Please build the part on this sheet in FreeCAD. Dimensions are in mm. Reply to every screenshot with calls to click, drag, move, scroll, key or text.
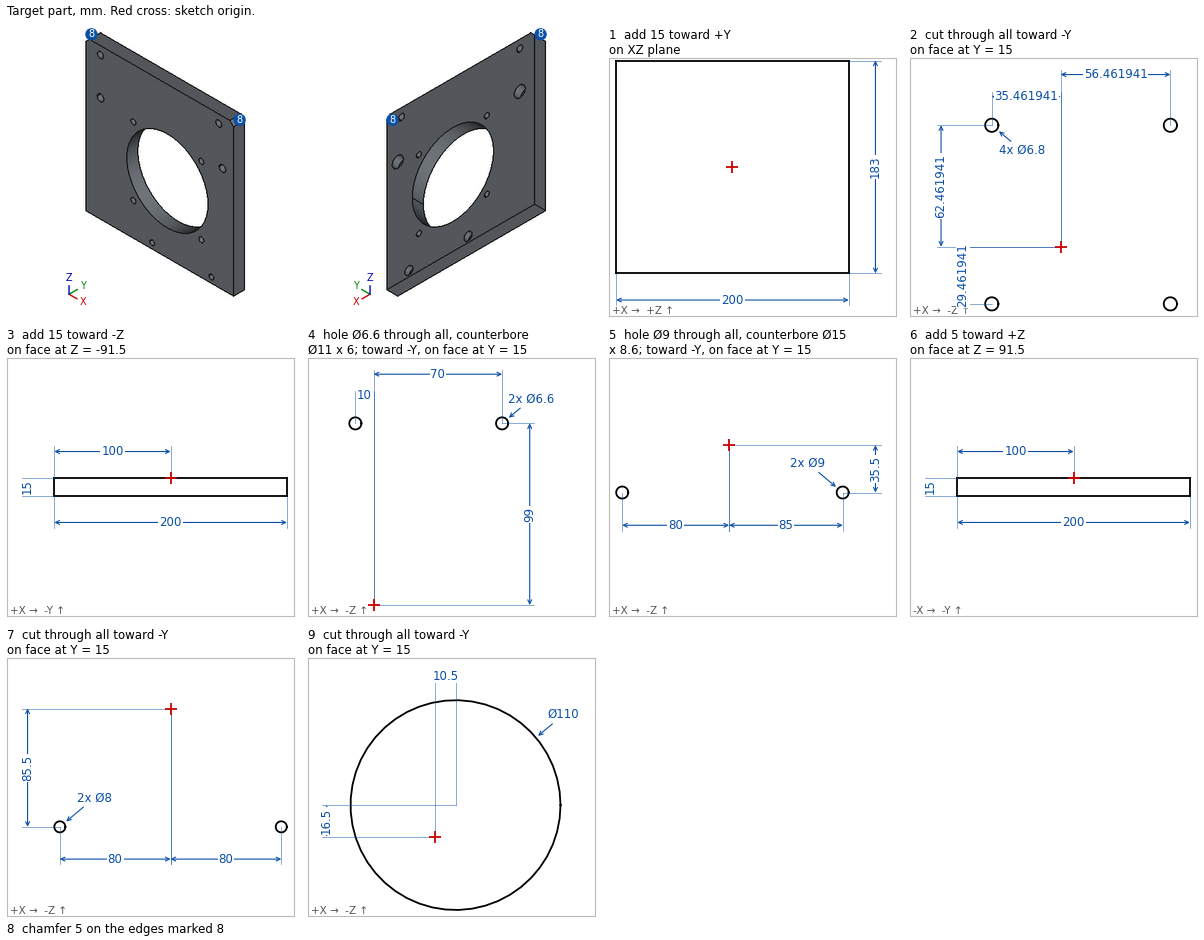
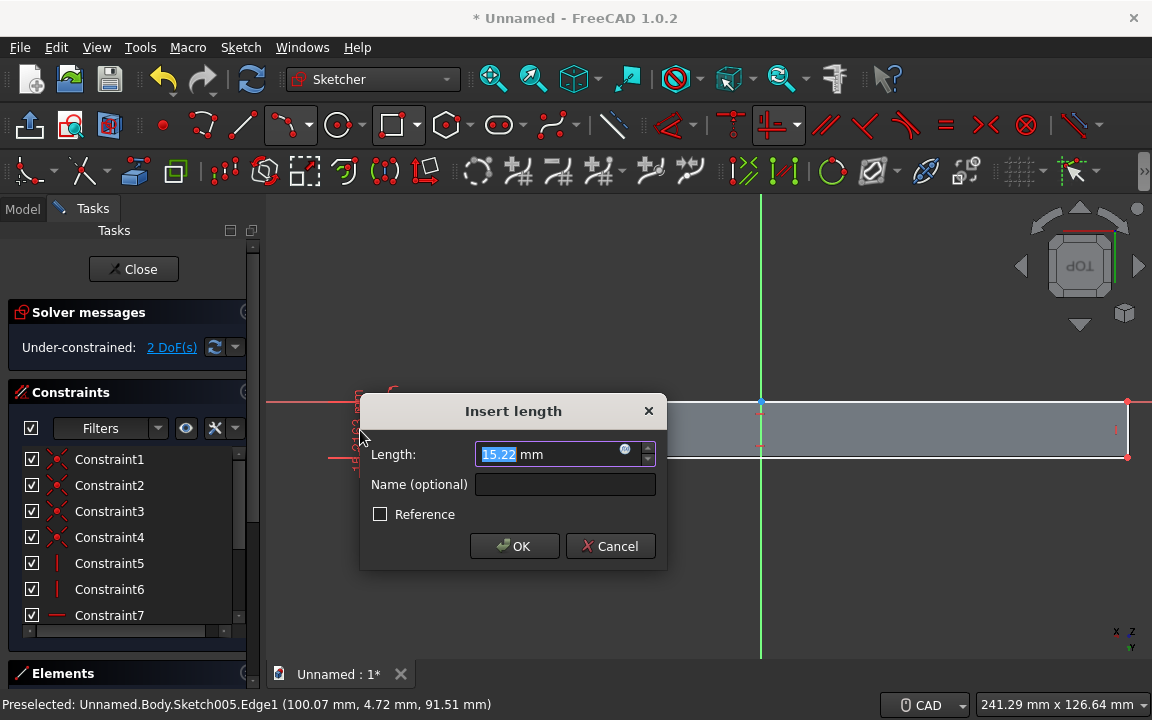
text(15)
key(Return)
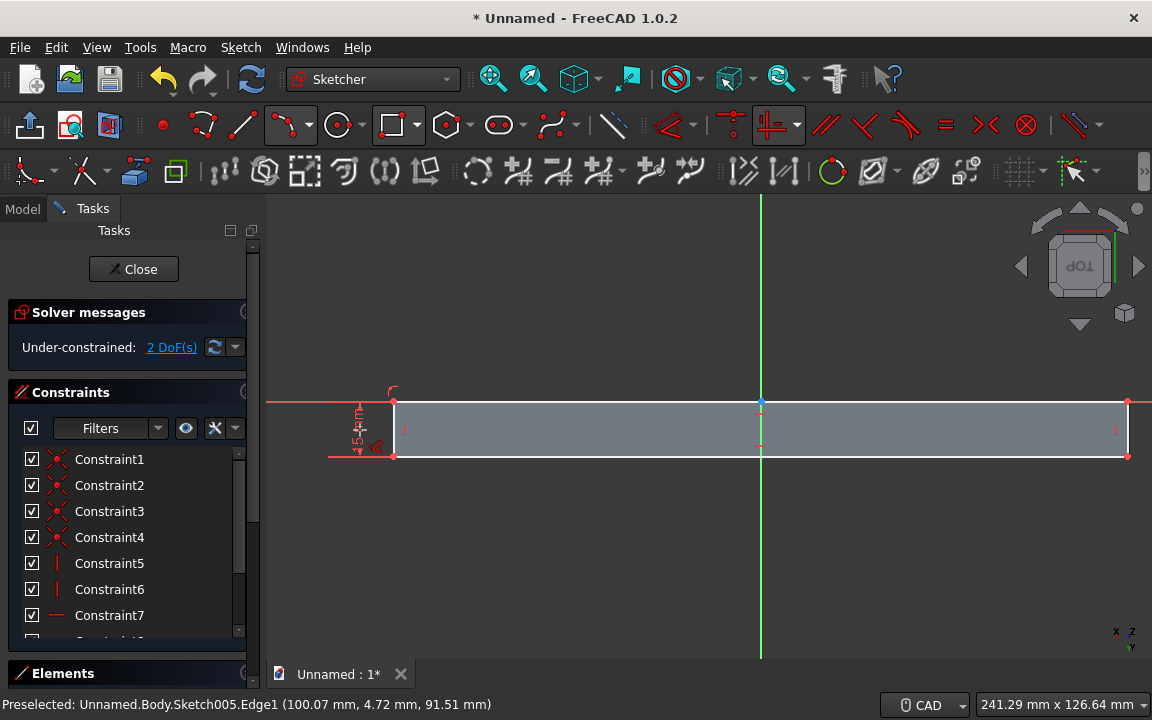
click(614, 457)
click(690, 491)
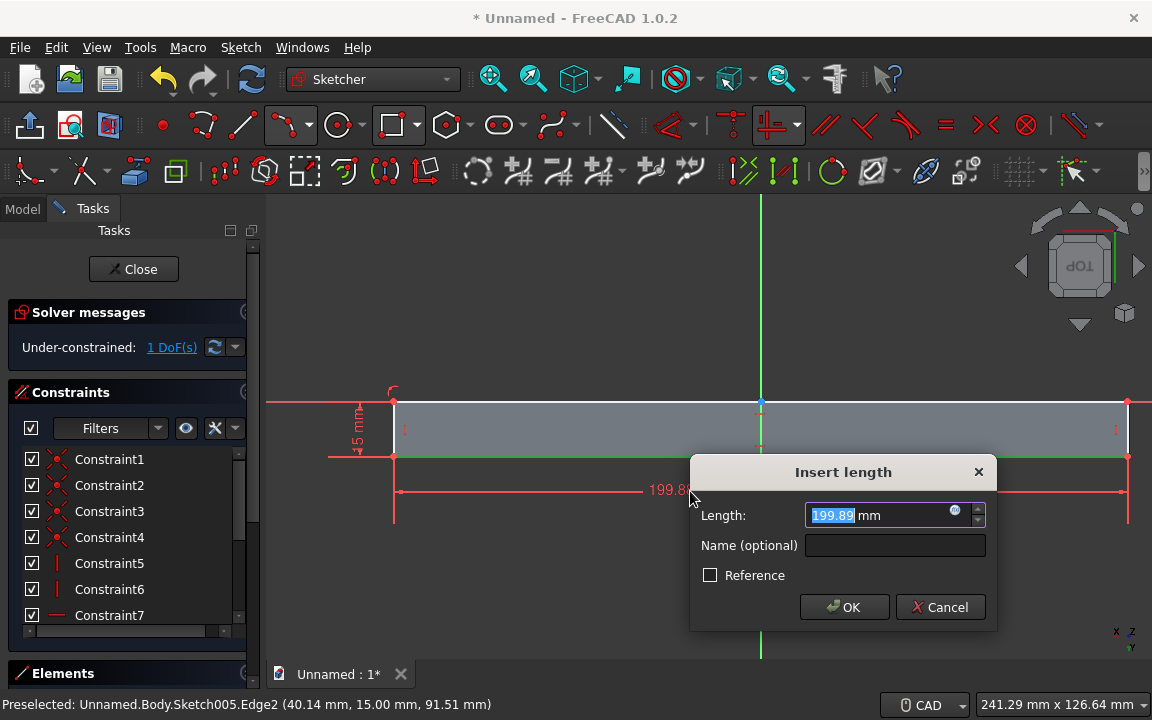
text(200)
key(Return)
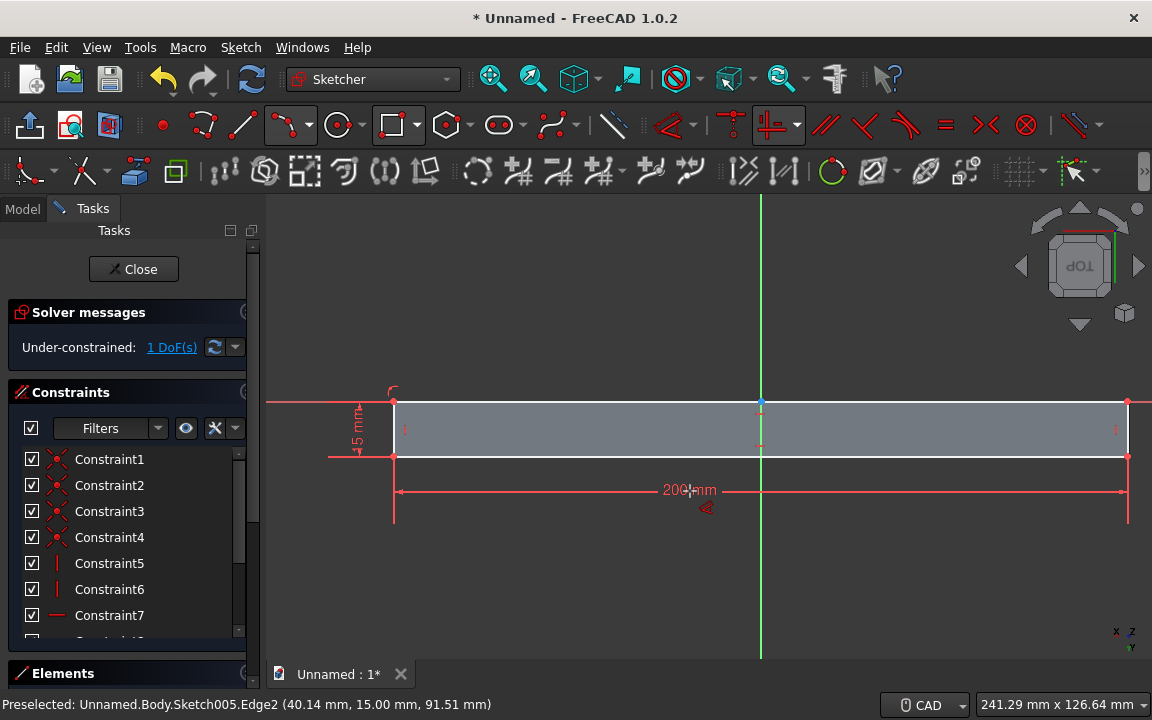
click(394, 402)
click(577, 368)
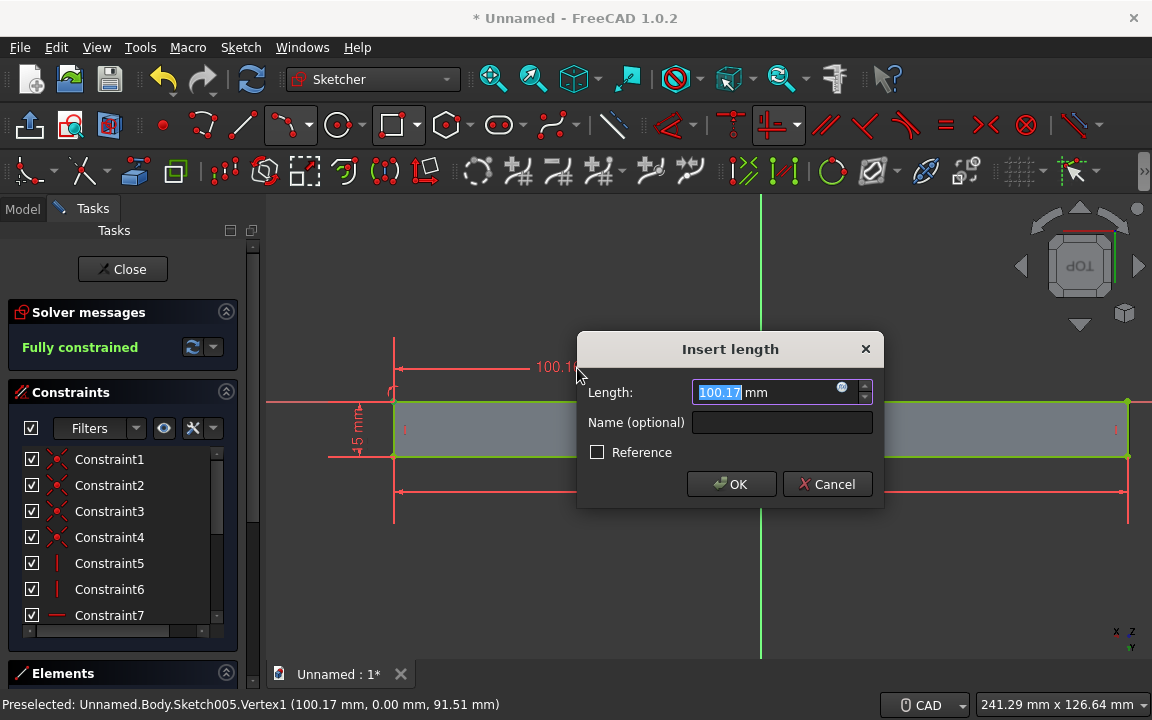
text(100)
key(Return)
key(Escape)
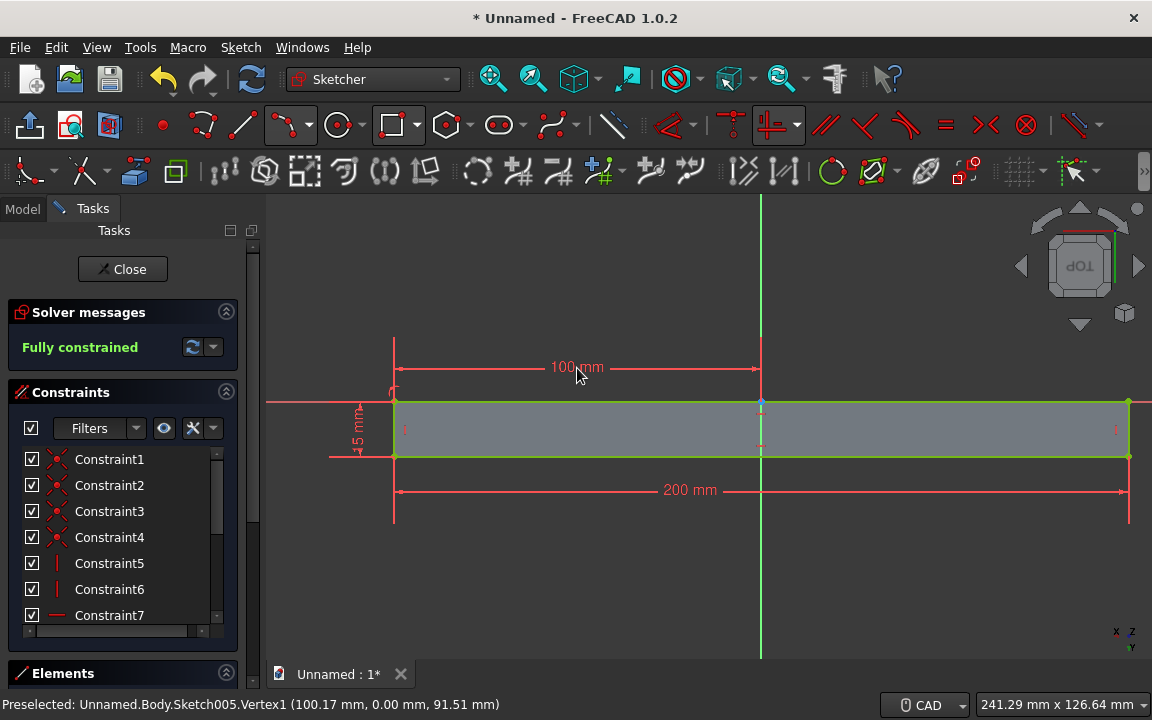
click(123, 269)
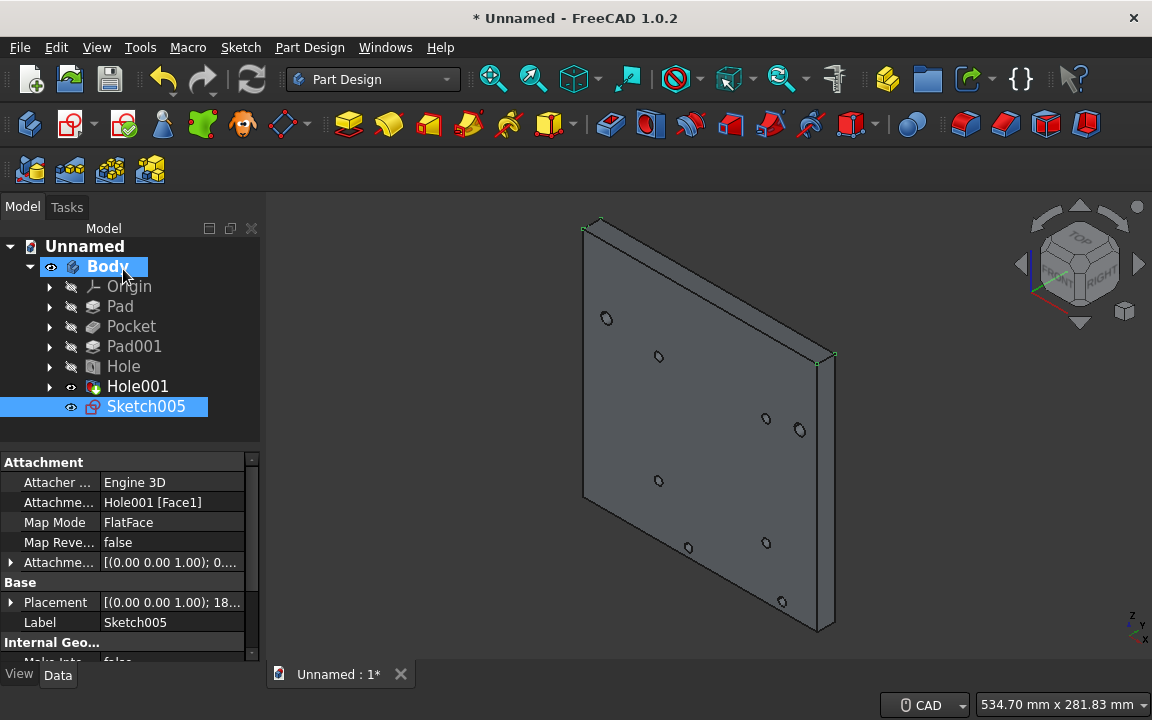
click(350, 124)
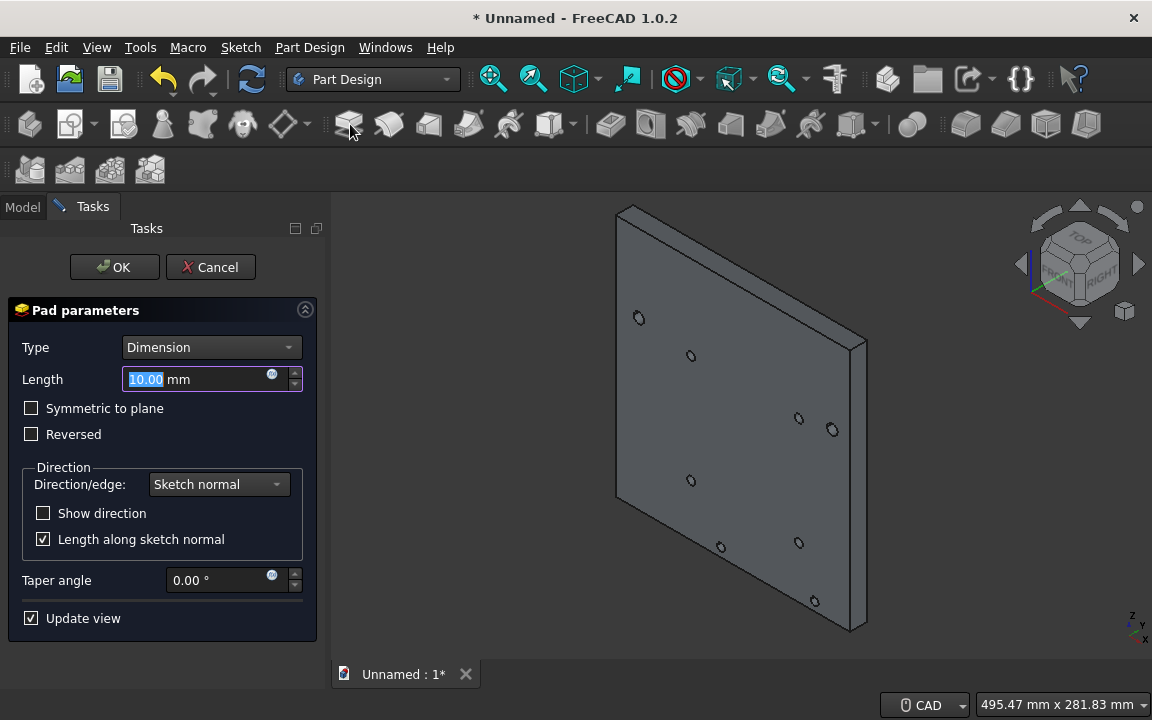
text(5)
key(Tab)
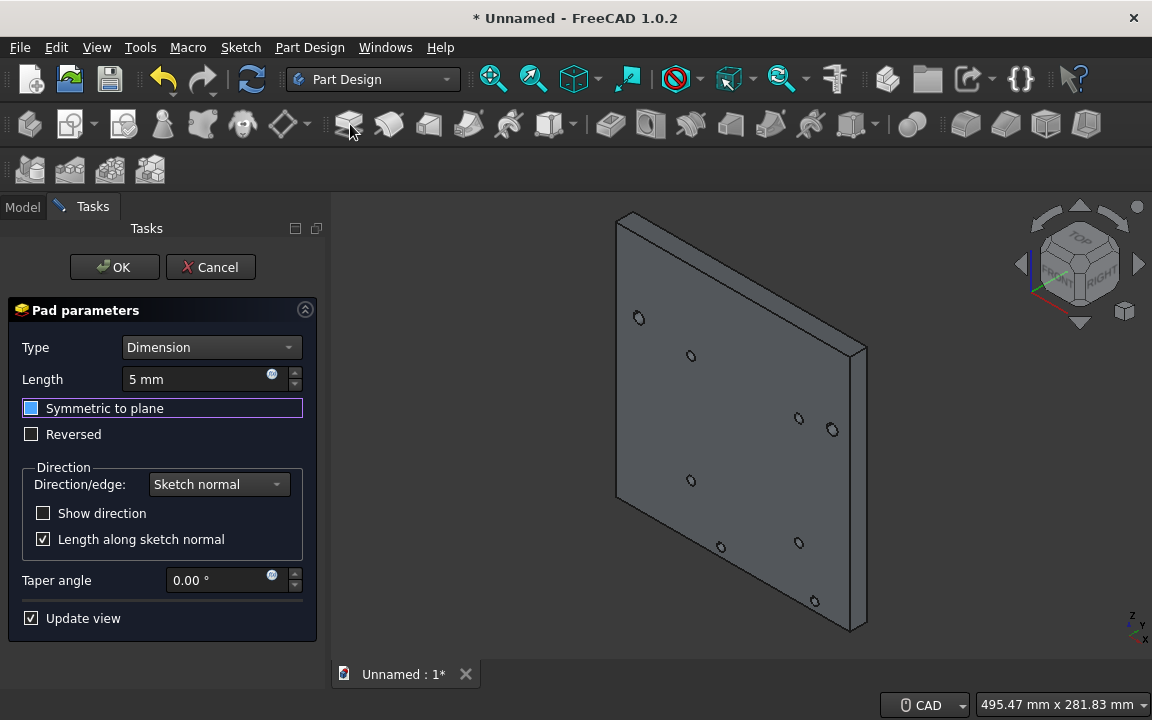
click(115, 267)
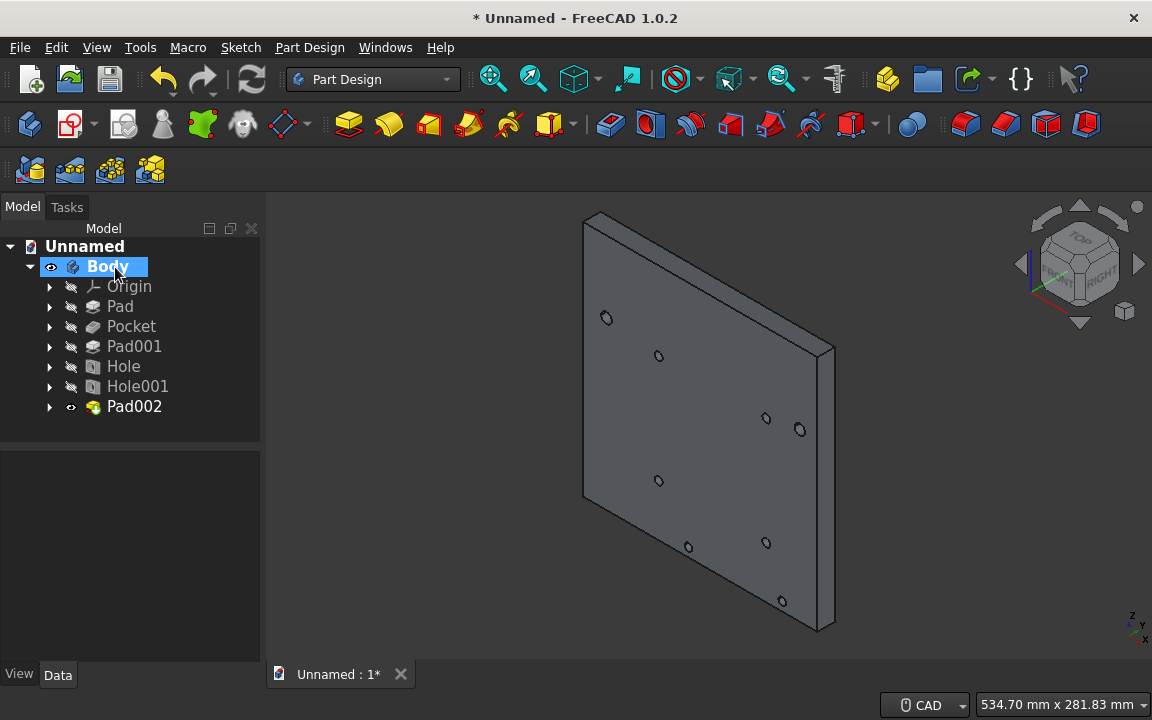
key(4)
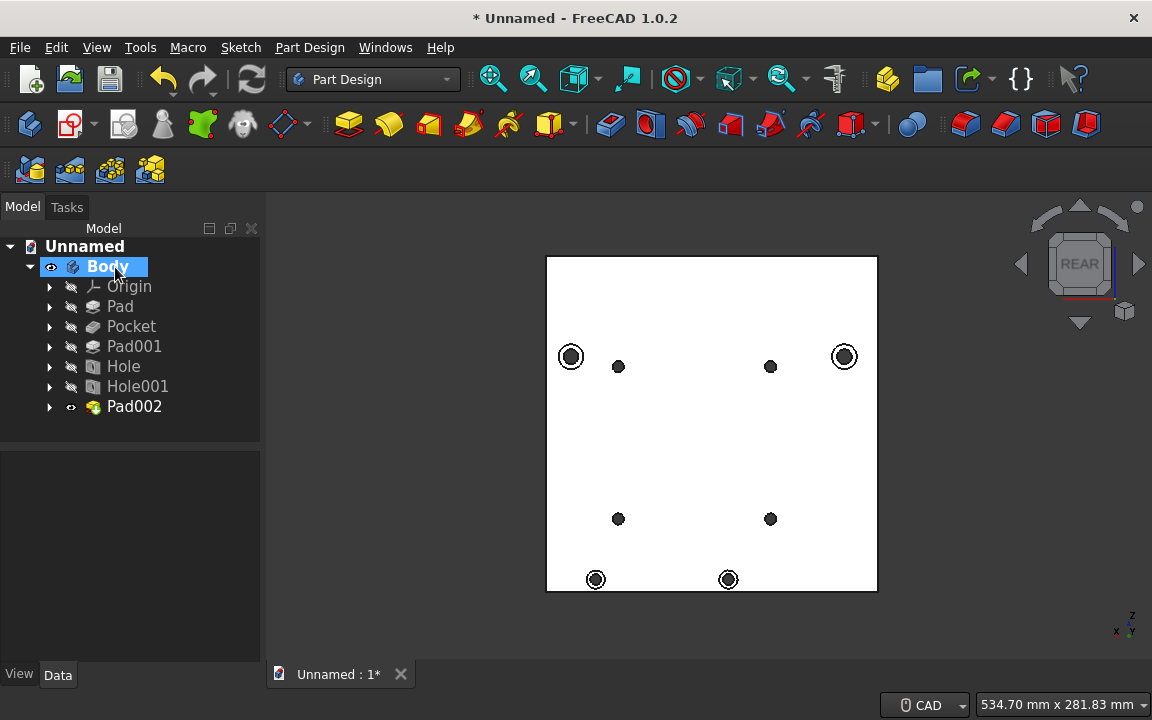
click(712, 423)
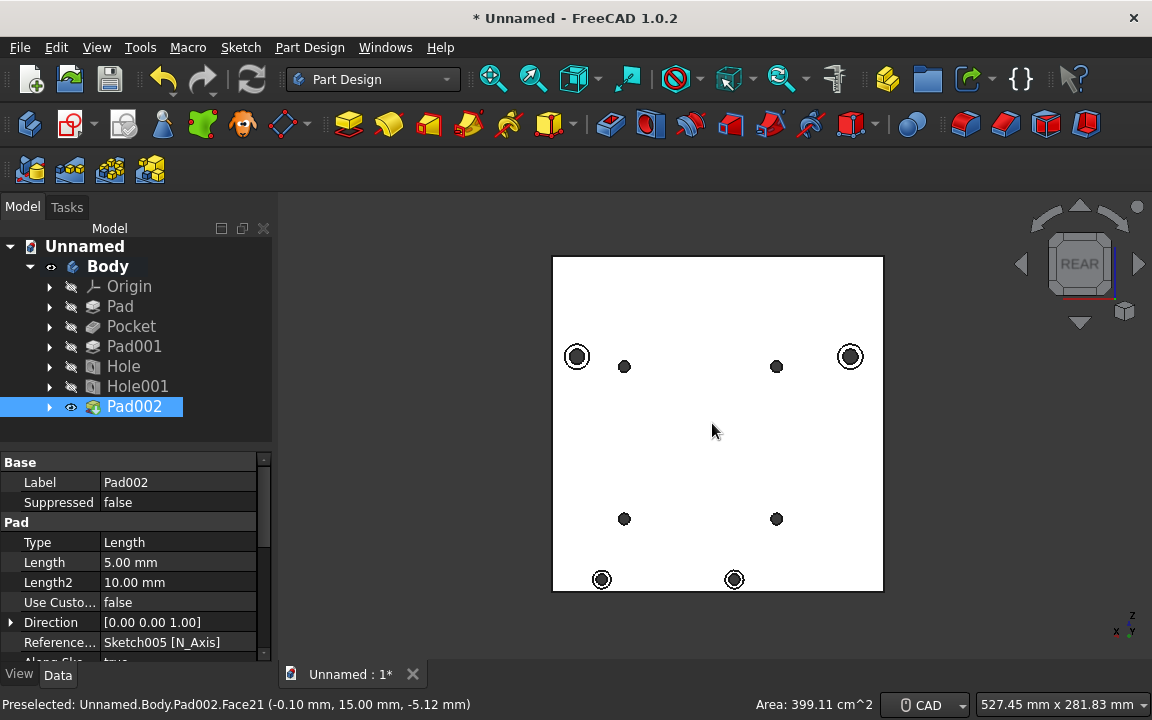
click(70, 124)